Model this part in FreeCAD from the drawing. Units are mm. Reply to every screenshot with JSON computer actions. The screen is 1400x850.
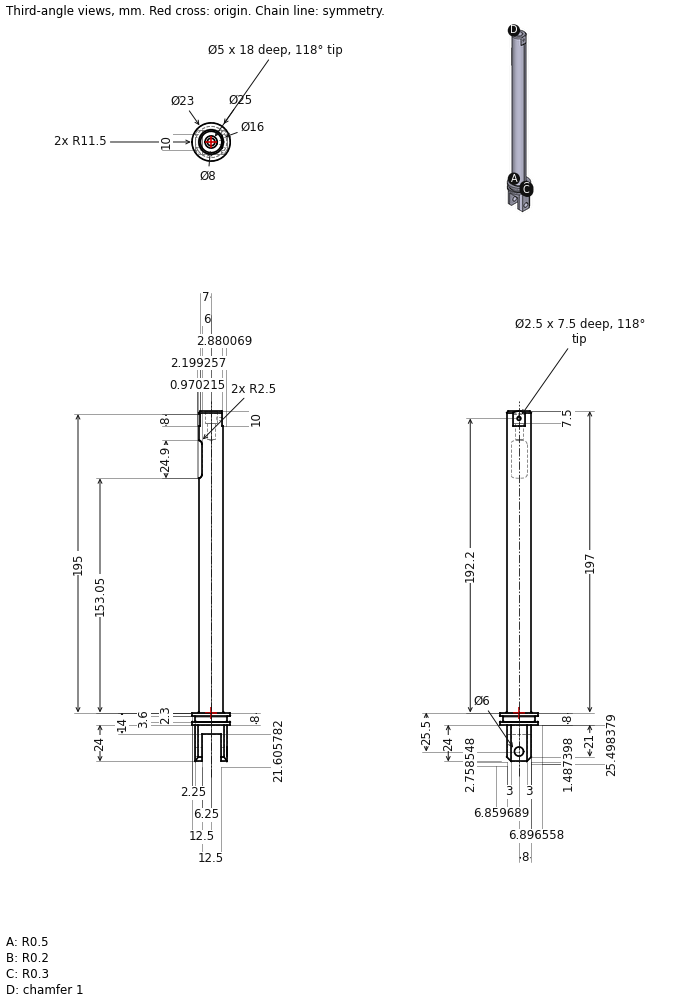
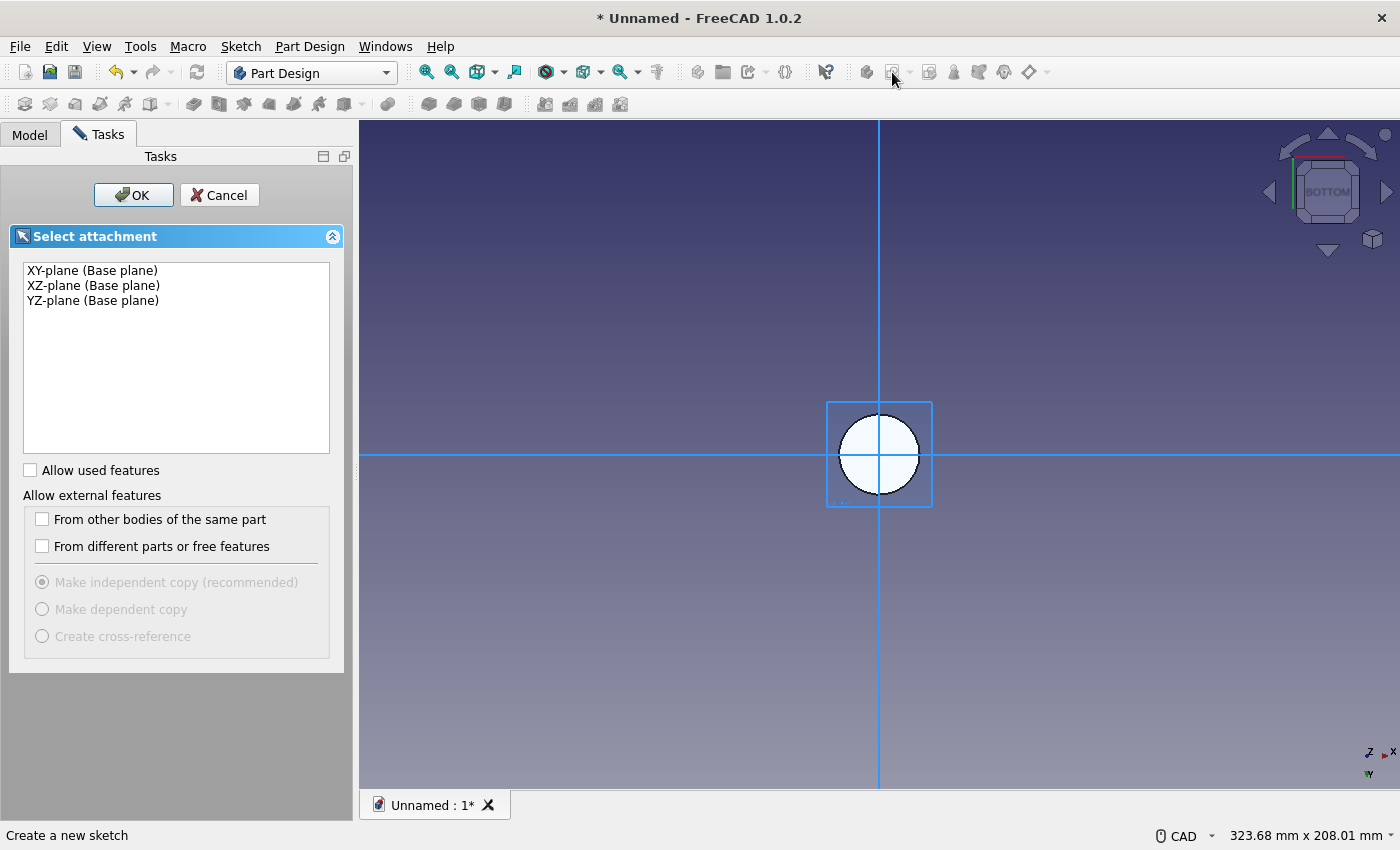
{"action": "left_click", "coordinate": [84, 286]}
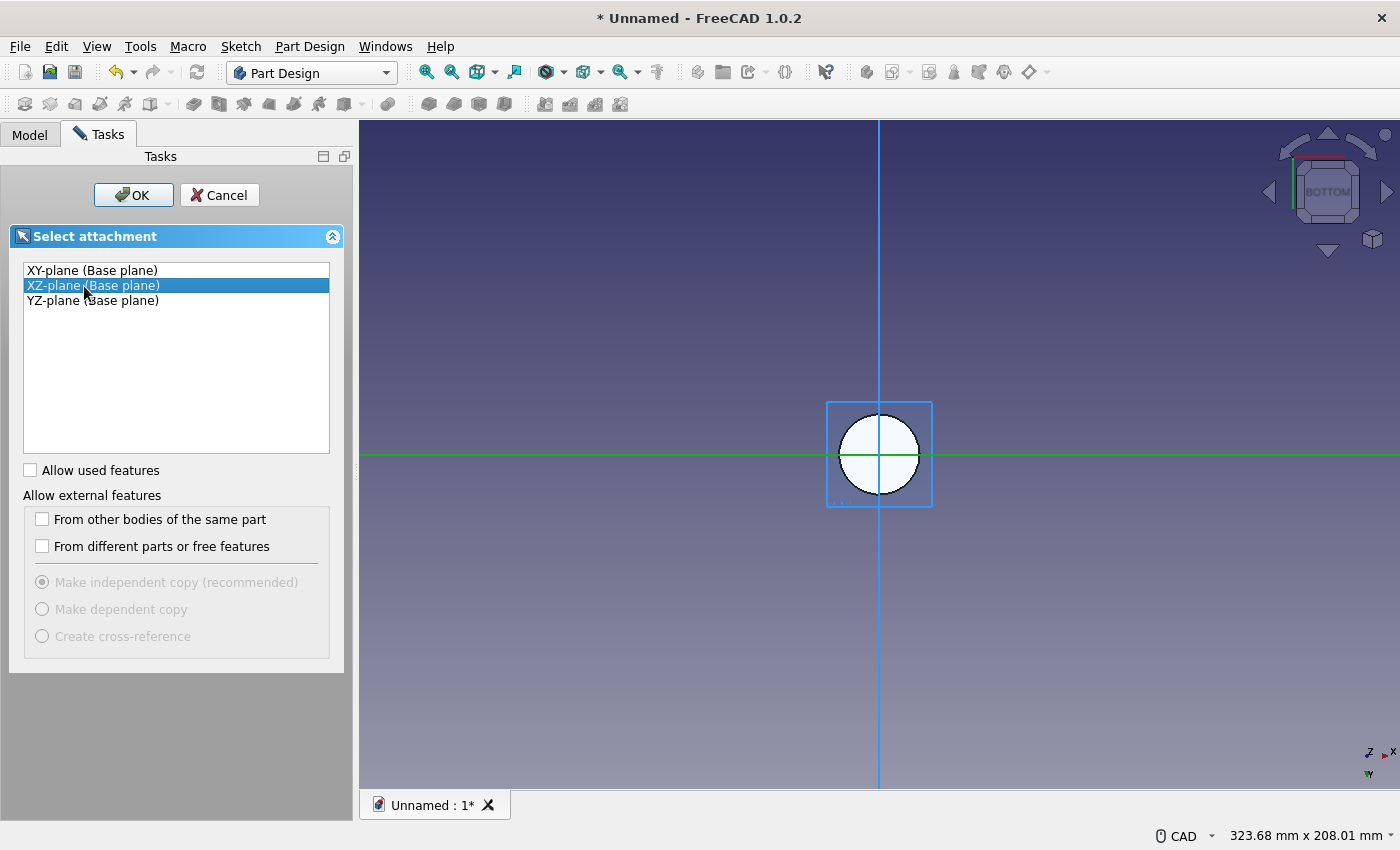
{"action": "left_click", "coordinate": [134, 195]}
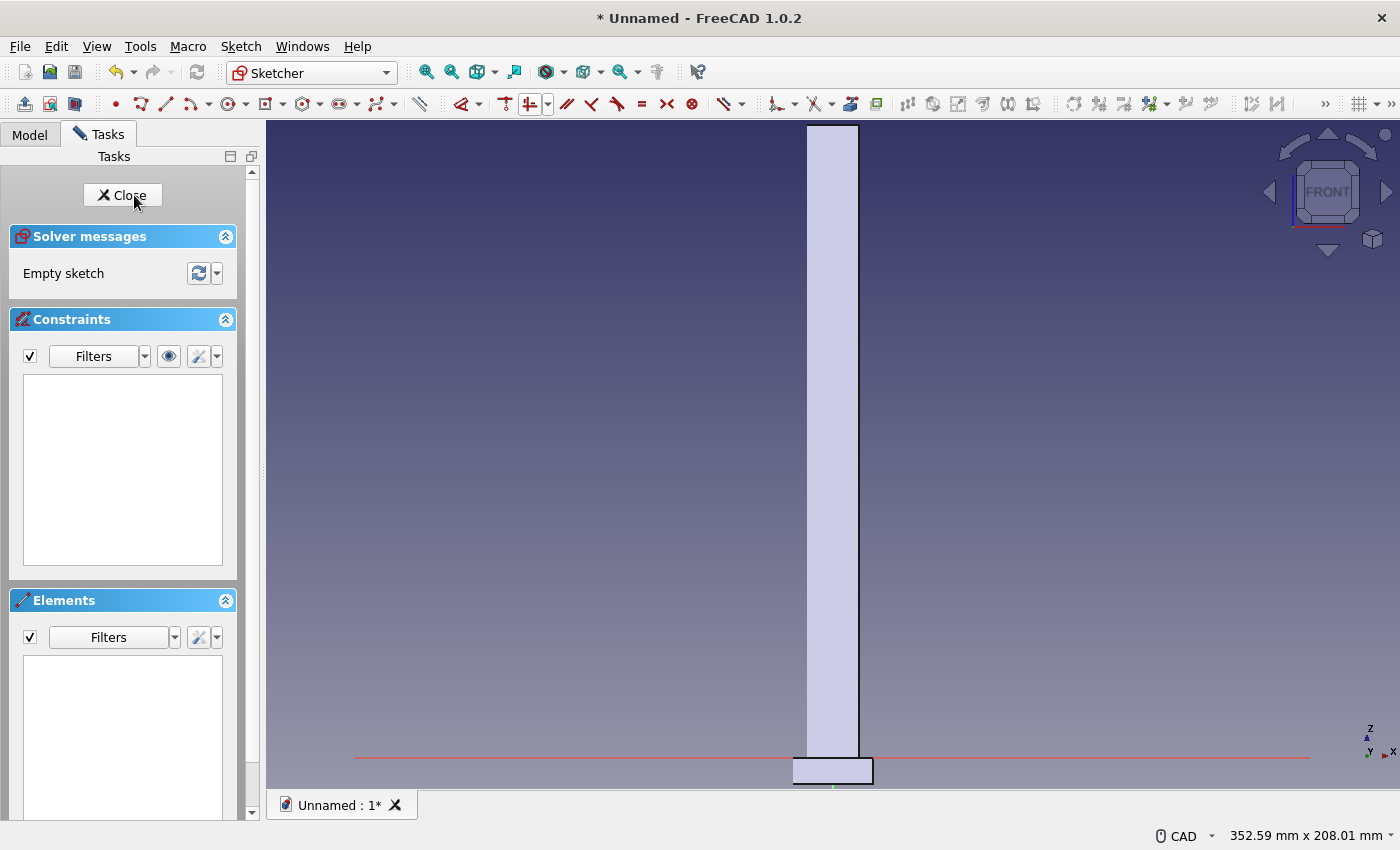
{"action": "left_click", "coordinate": [75, 104]}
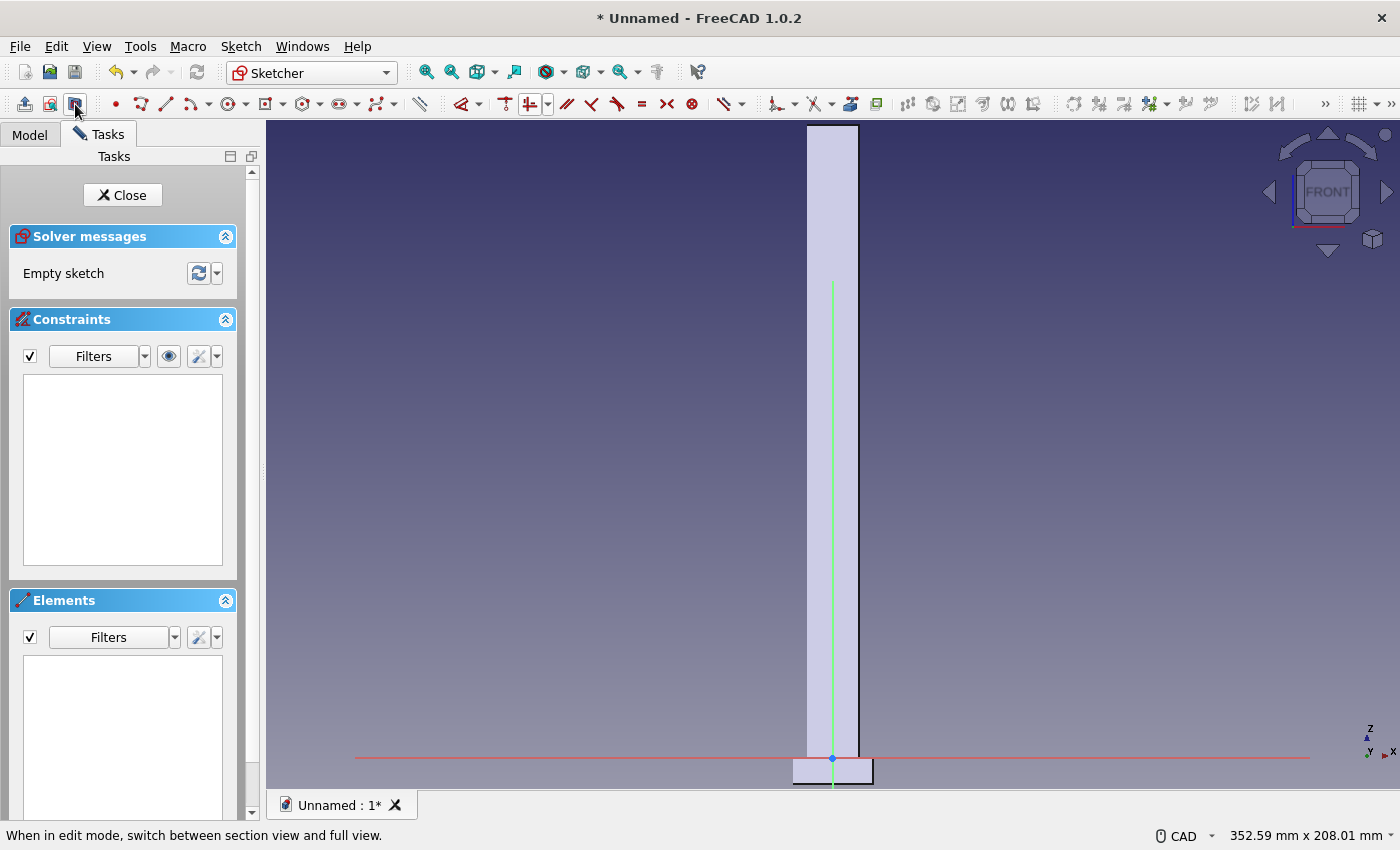
{"action": "scroll", "coordinate": [764, 454], "scroll_direction": "down", "scroll_amount": 5}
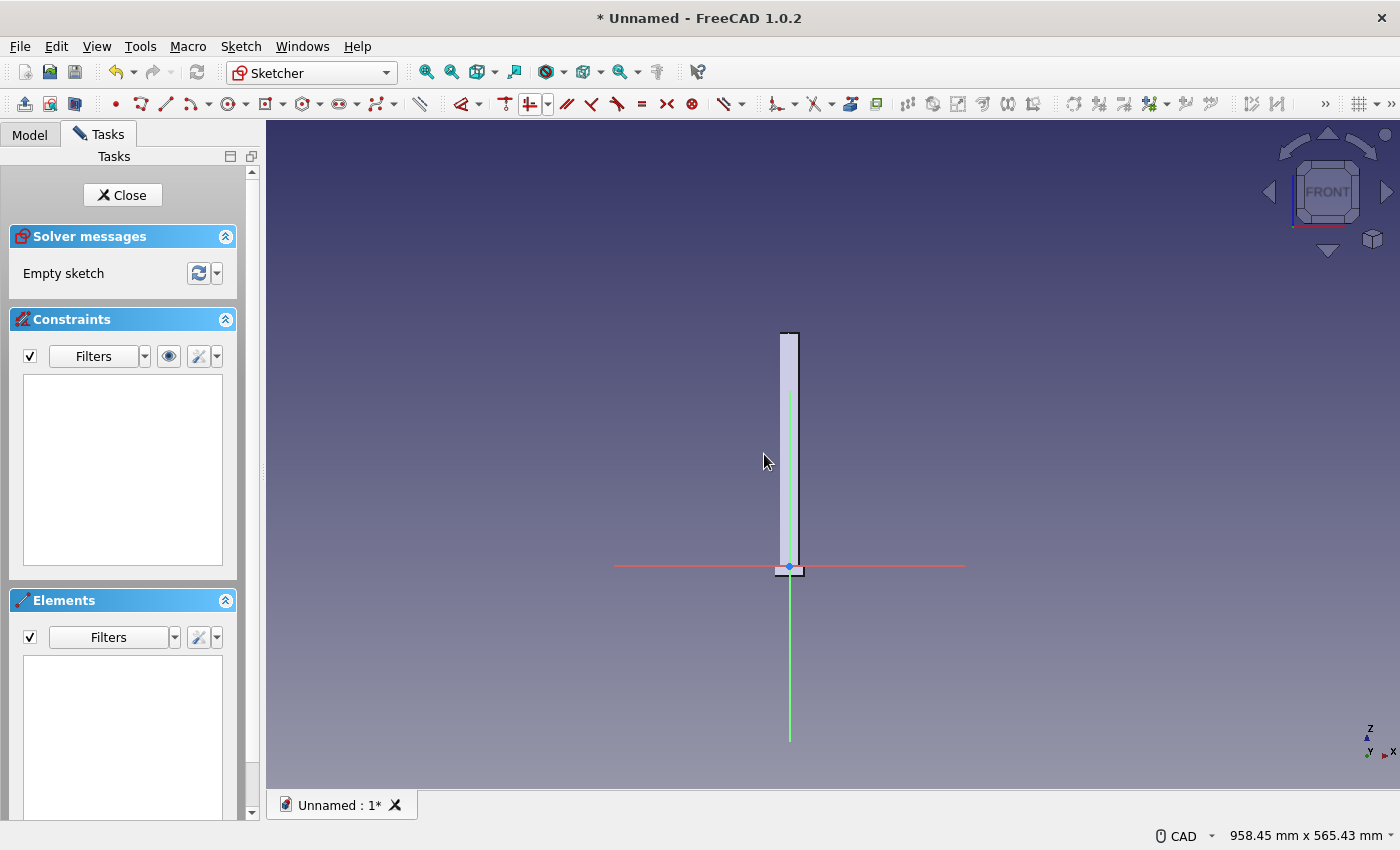
{"action": "scroll", "coordinate": [777, 577], "scroll_direction": "up", "scroll_amount": 15}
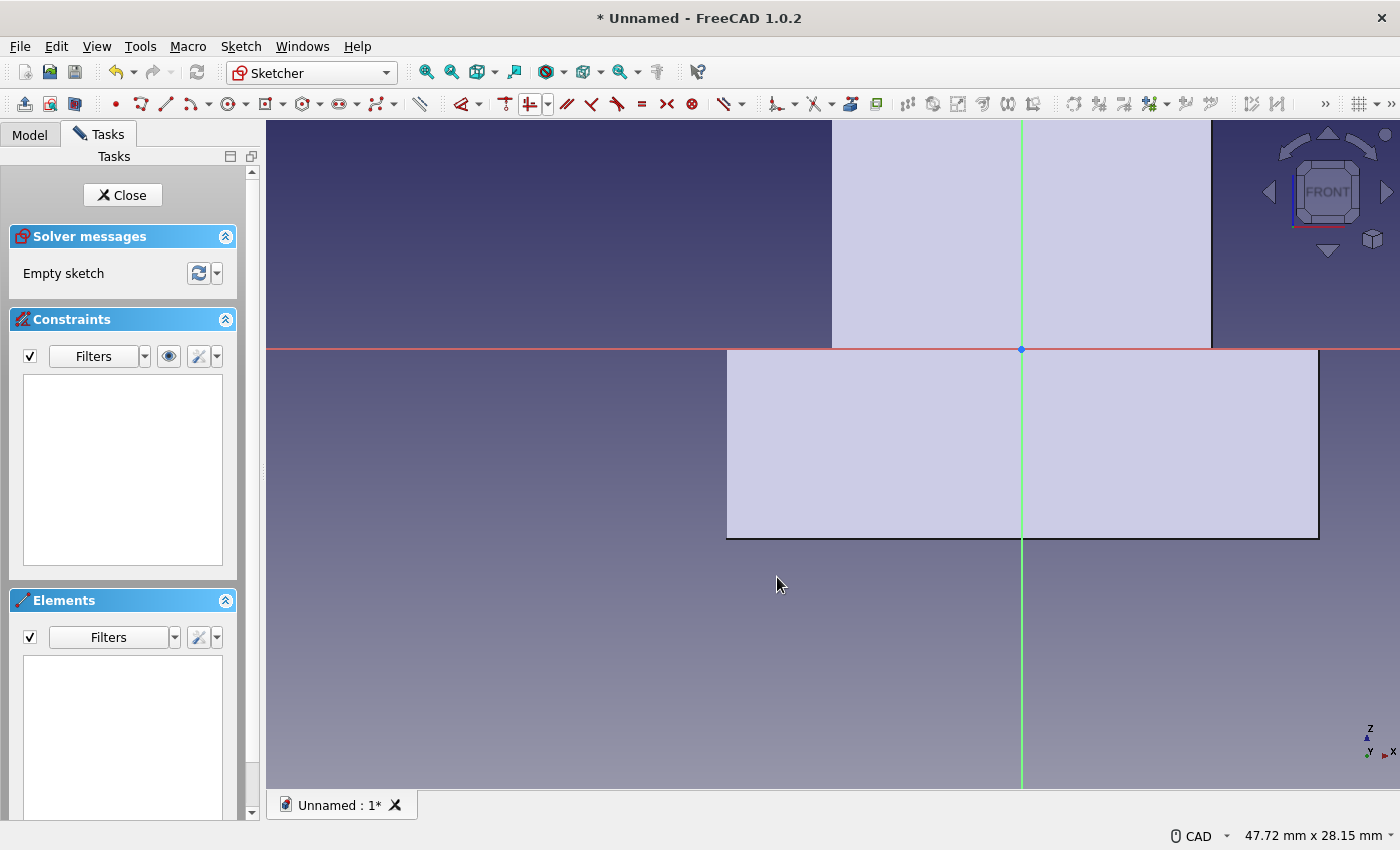
{"action": "scroll", "coordinate": [748, 445], "scroll_direction": "up", "scroll_amount": 8}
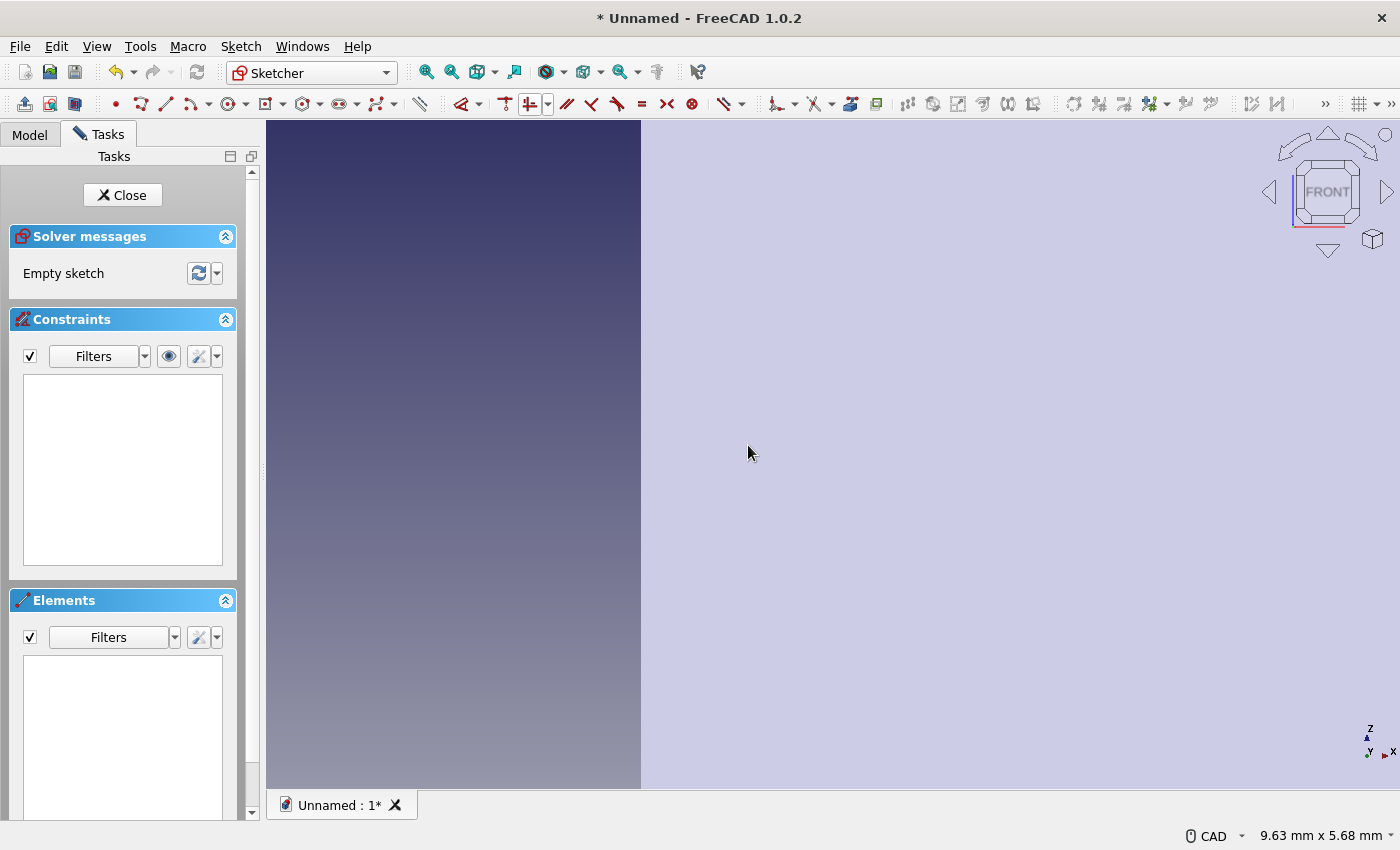
{"action": "left_click", "coordinate": [282, 104]}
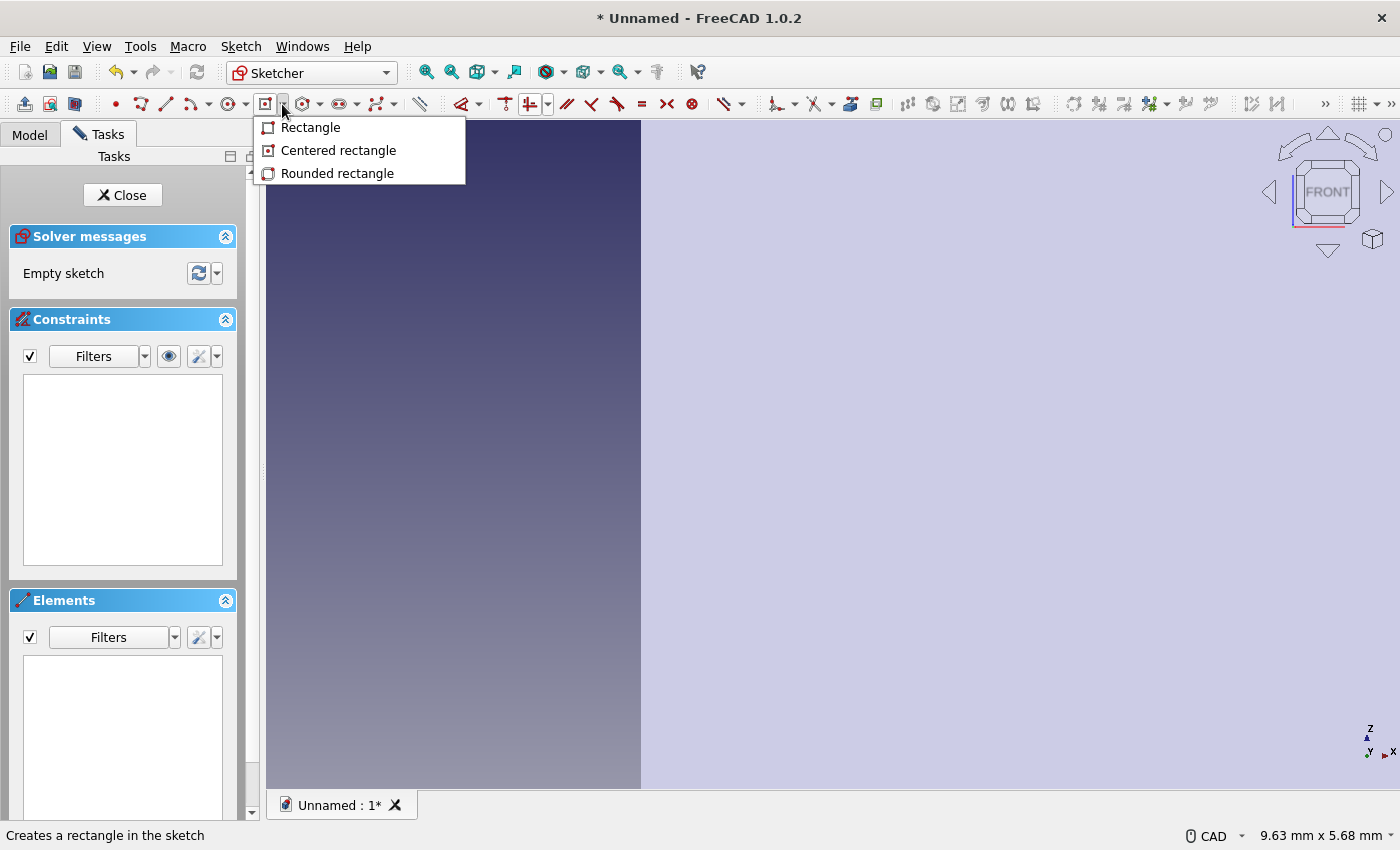
{"action": "left_click", "coordinate": [360, 128]}